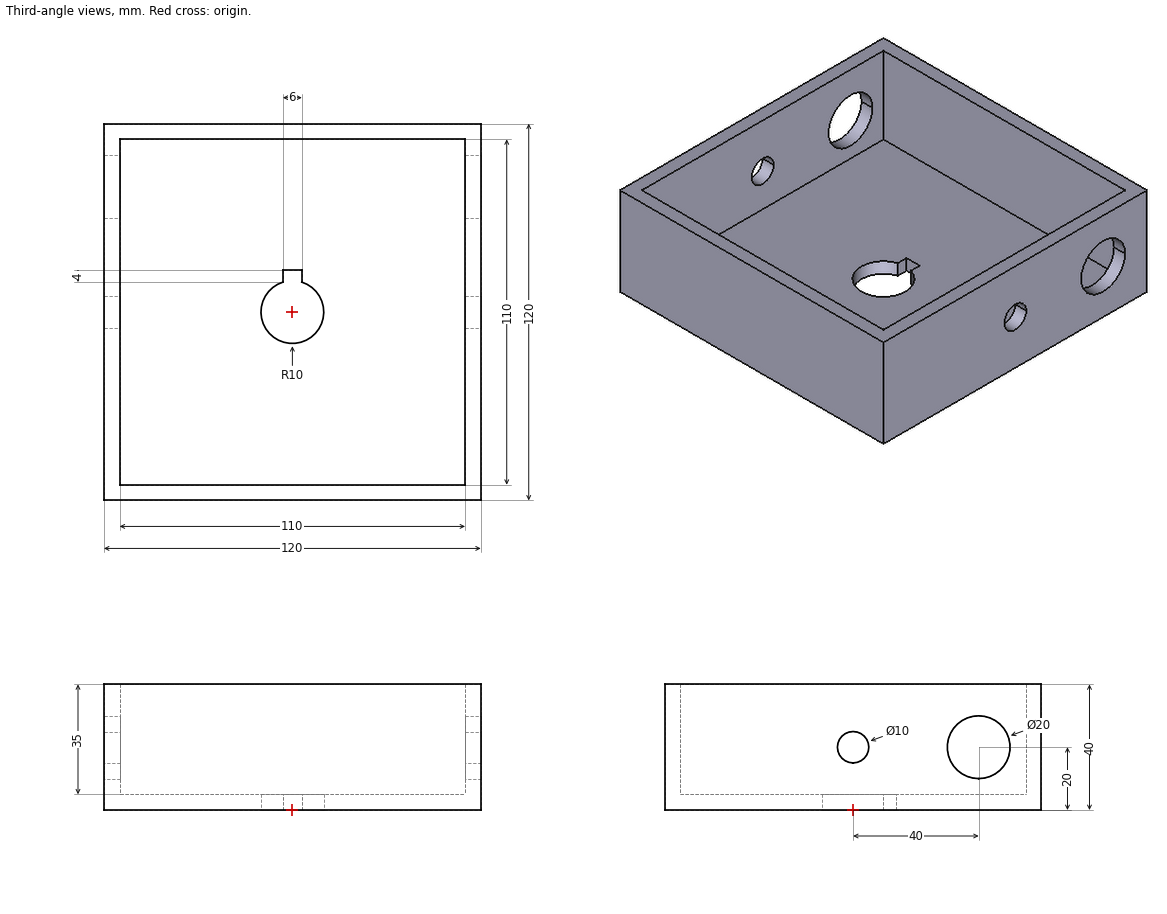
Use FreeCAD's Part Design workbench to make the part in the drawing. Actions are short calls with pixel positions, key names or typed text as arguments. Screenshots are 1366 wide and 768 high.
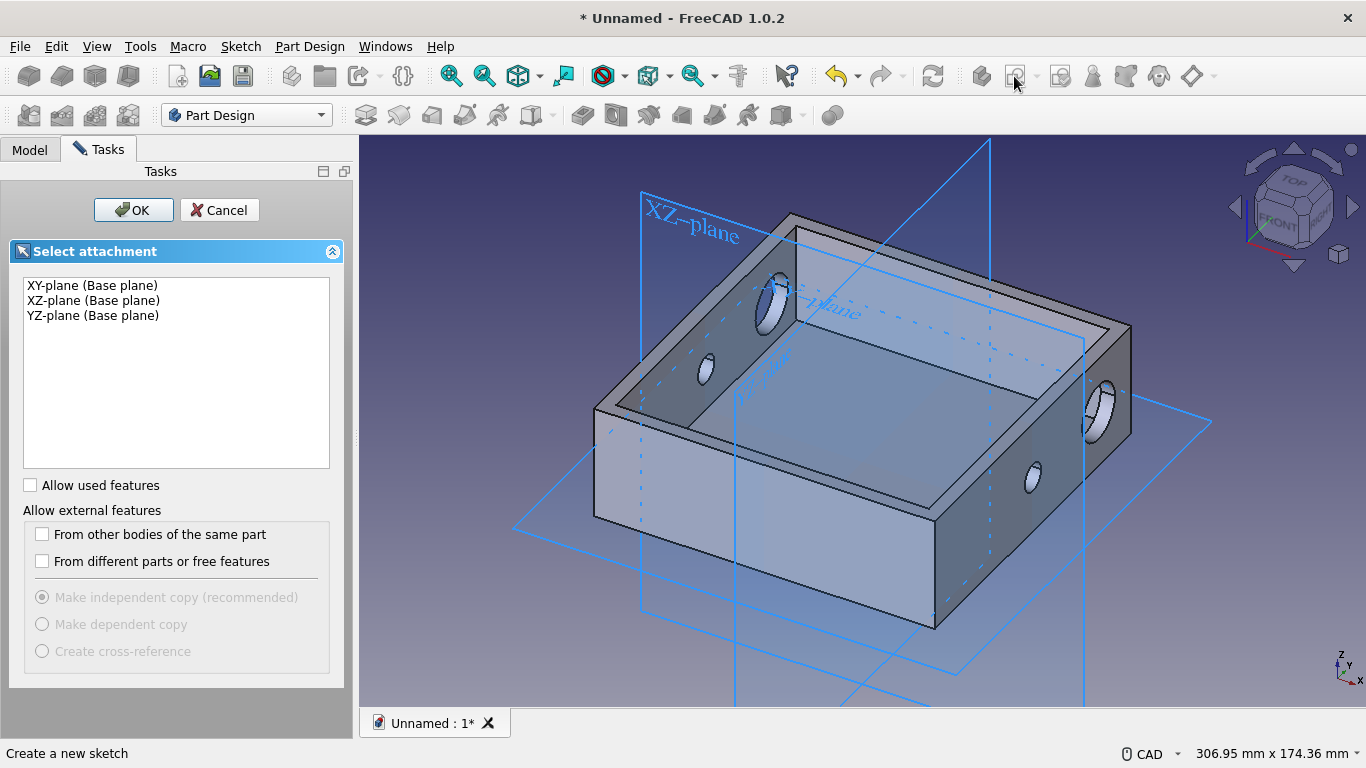
click(84, 286)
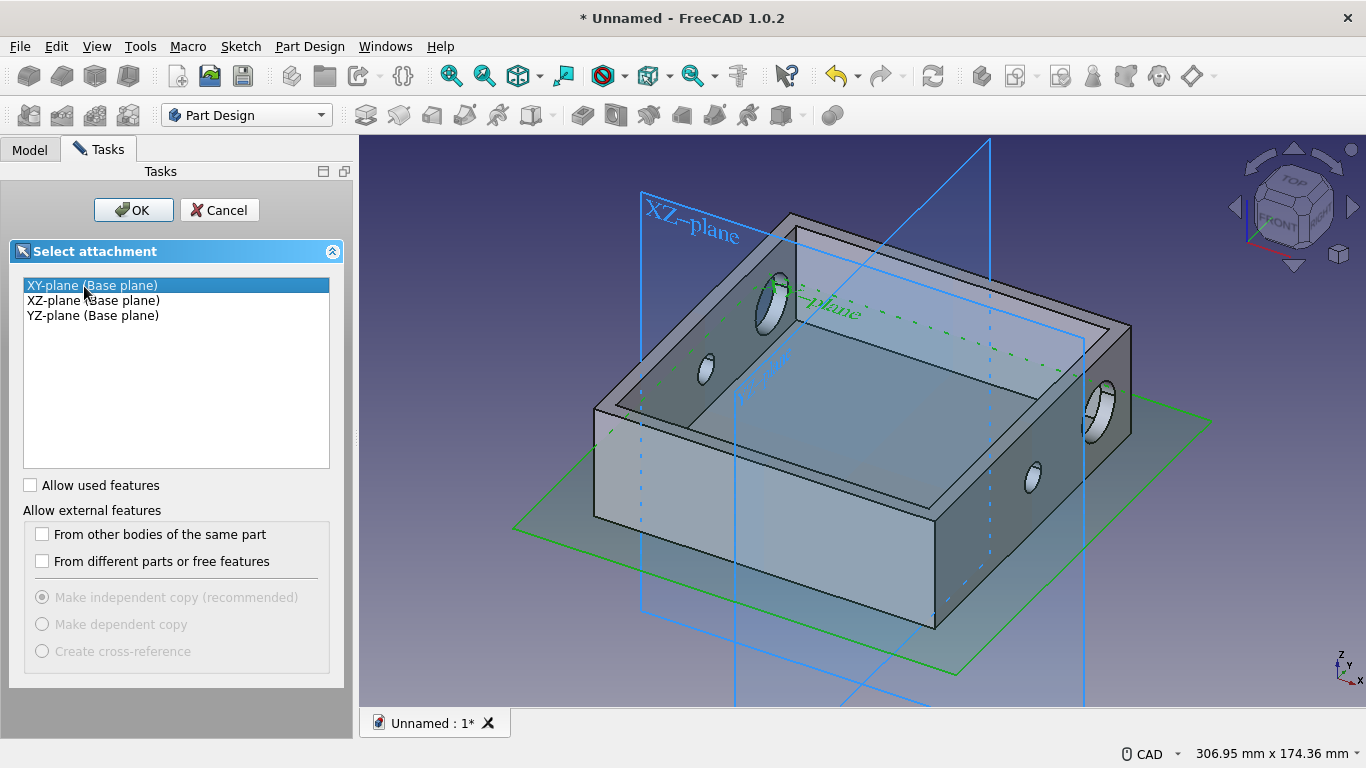
click(134, 210)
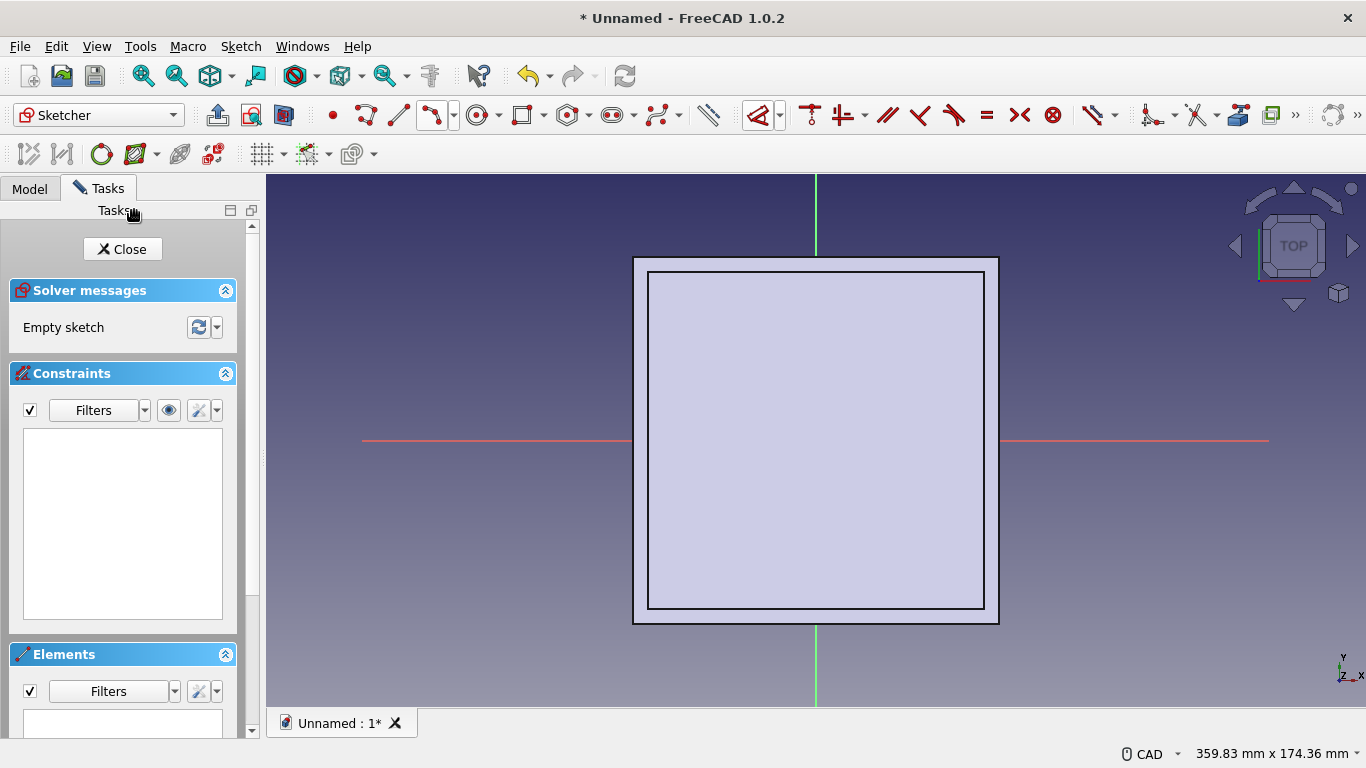
click(284, 116)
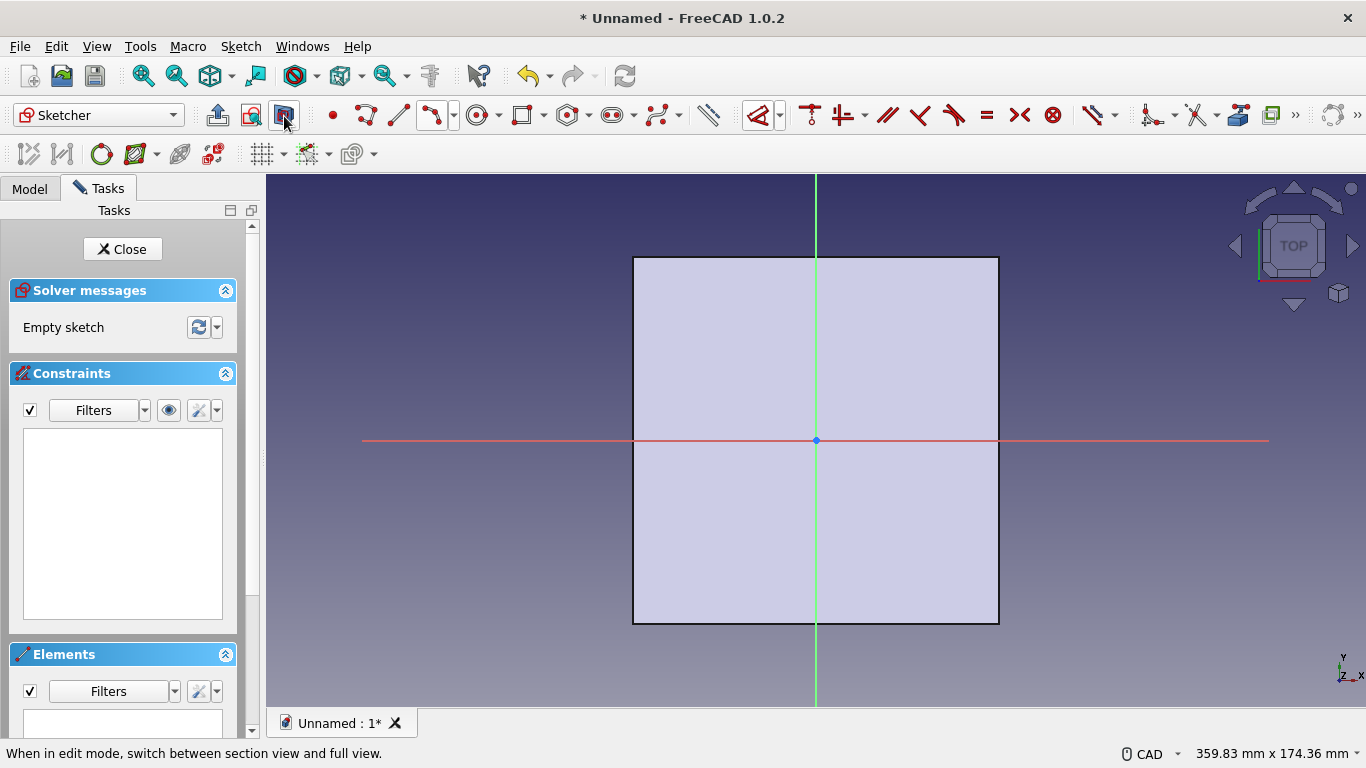
scroll(833, 434, up, 8)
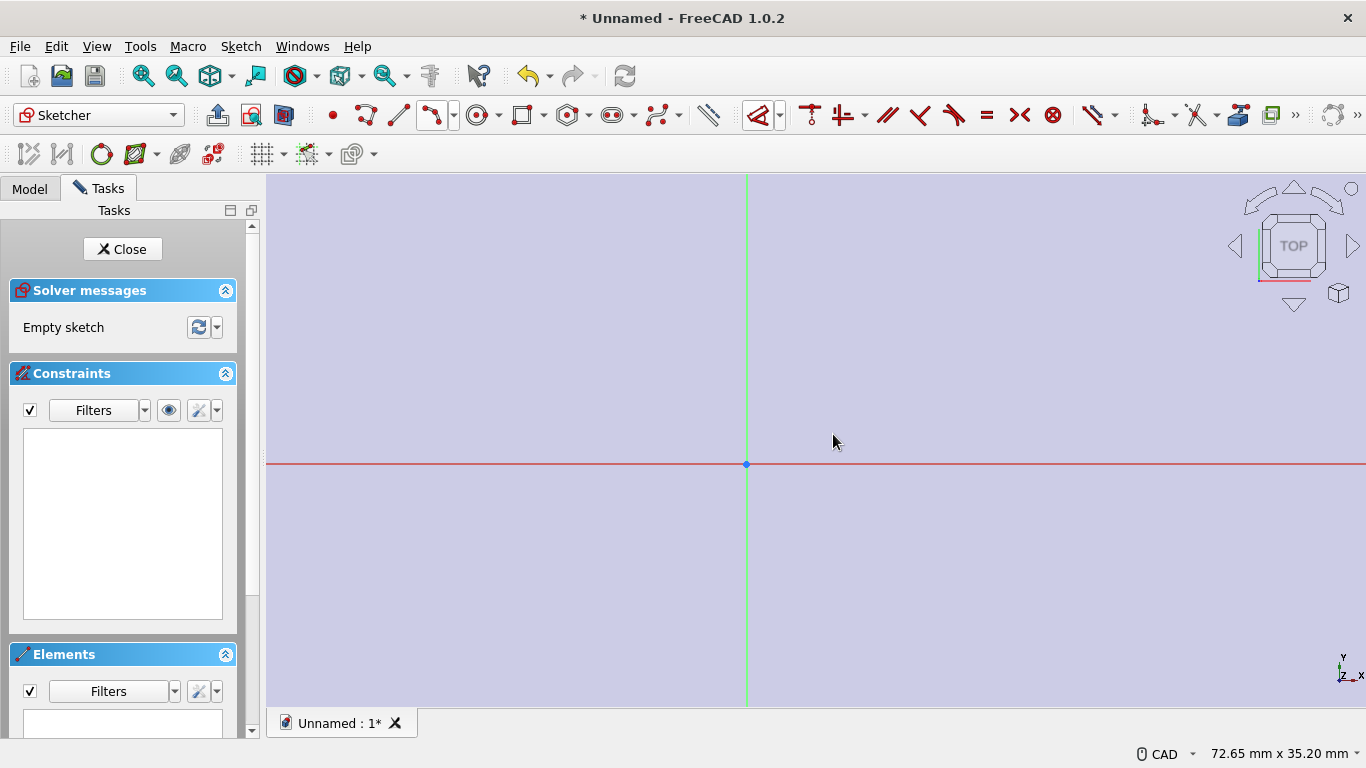
key(g)
key(m)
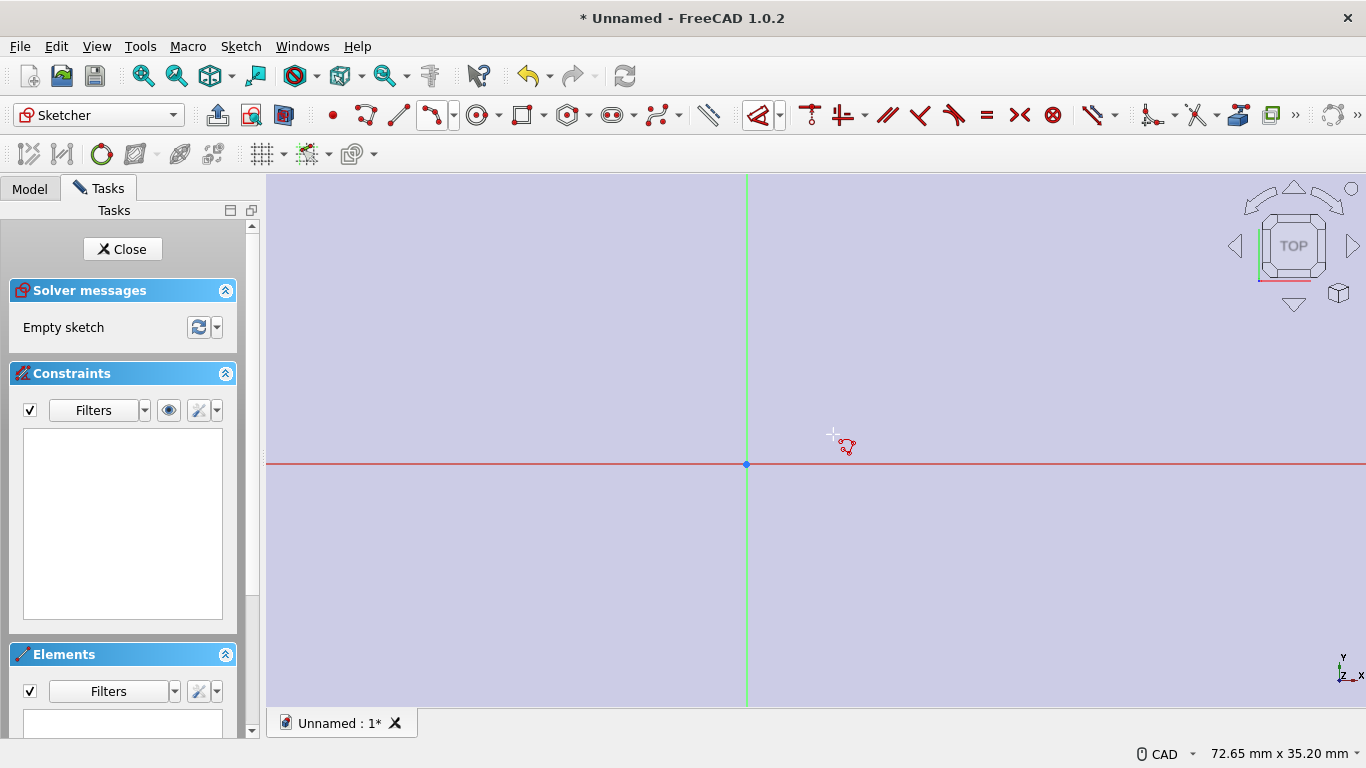
click(701, 320)
click(701, 259)
click(792, 259)
click(792, 320)
right_click(792, 320)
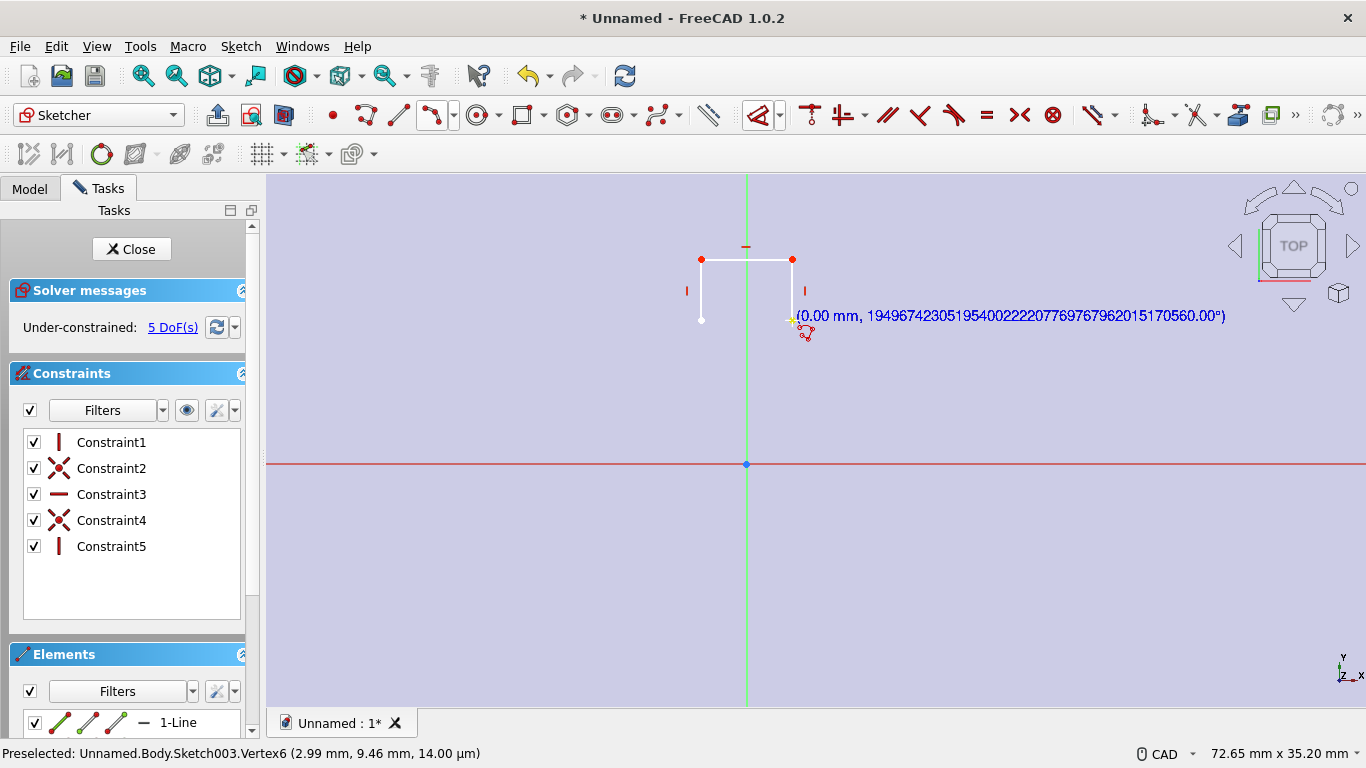
click(432, 116)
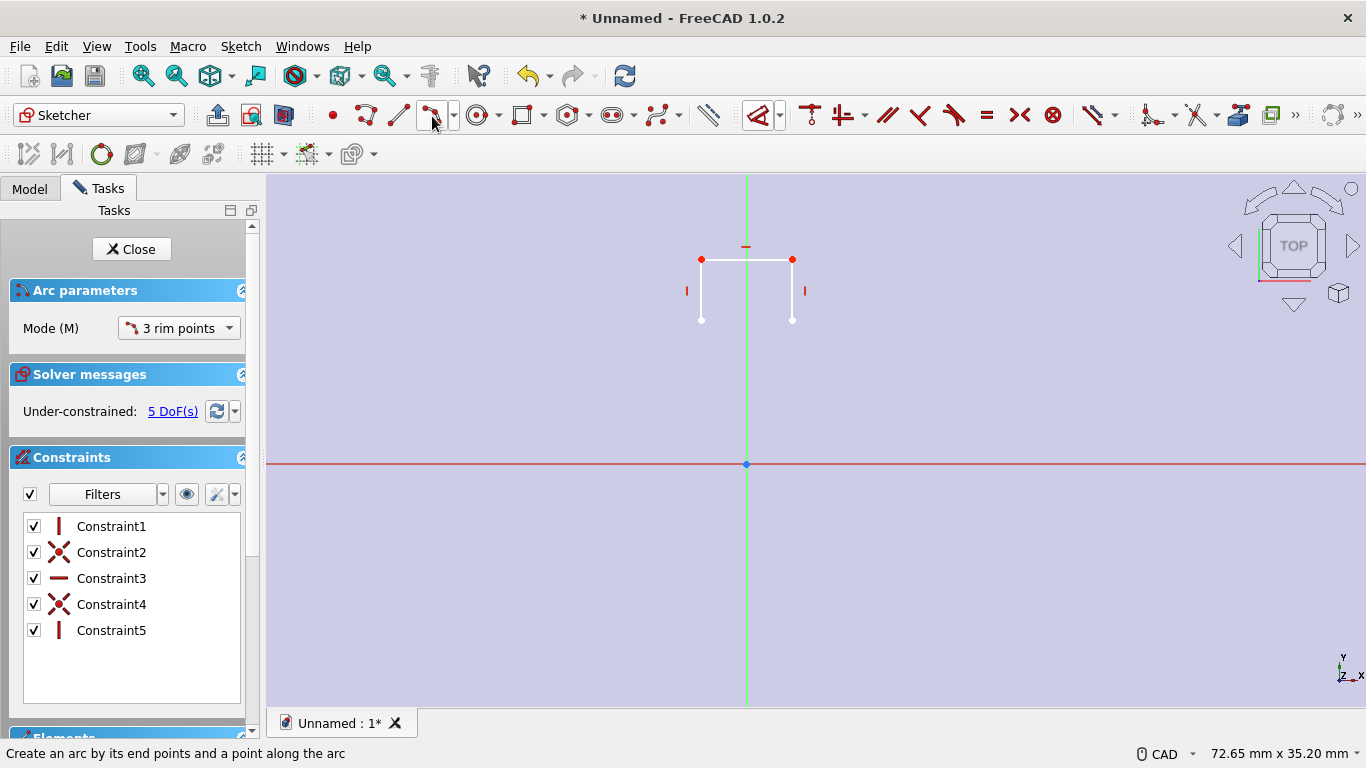
click(792, 321)
click(701, 321)
click(665, 592)
key(Escape)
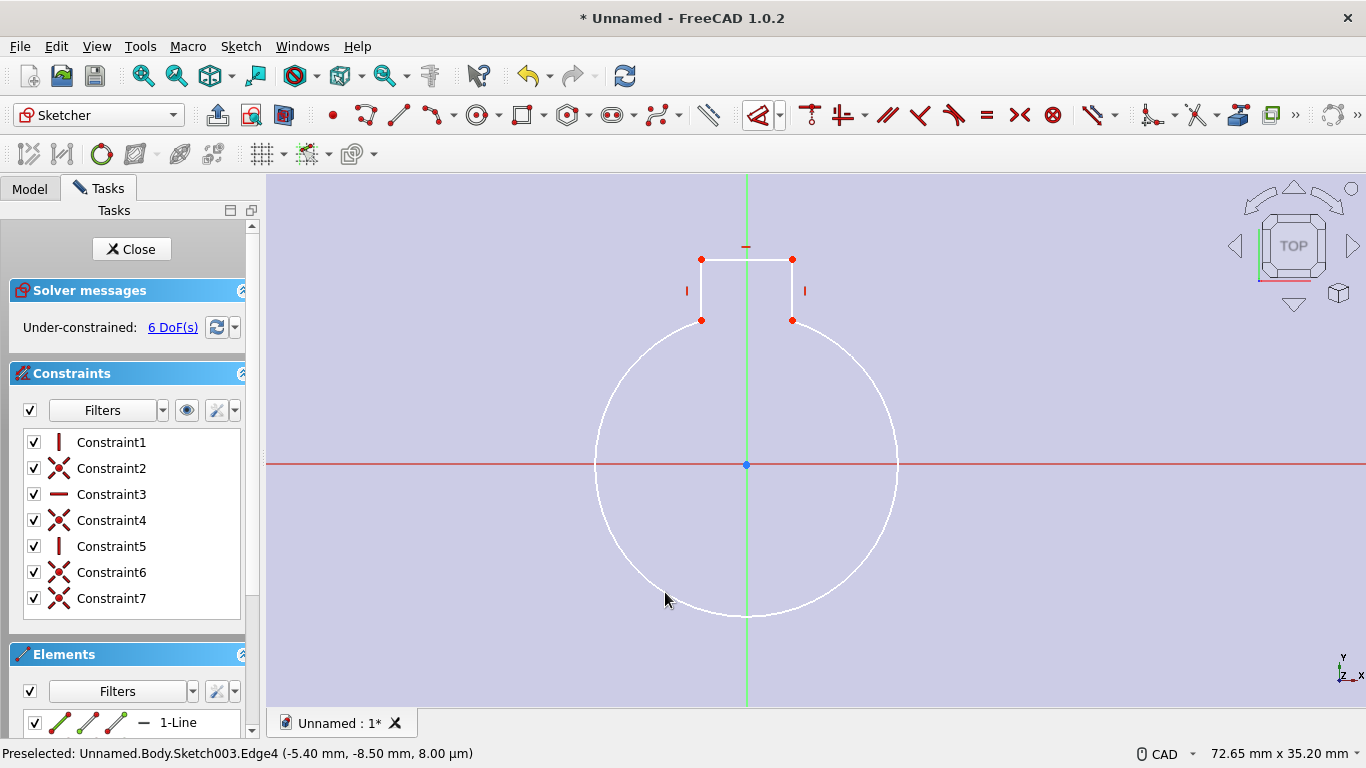
drag(737, 454, 757, 475)